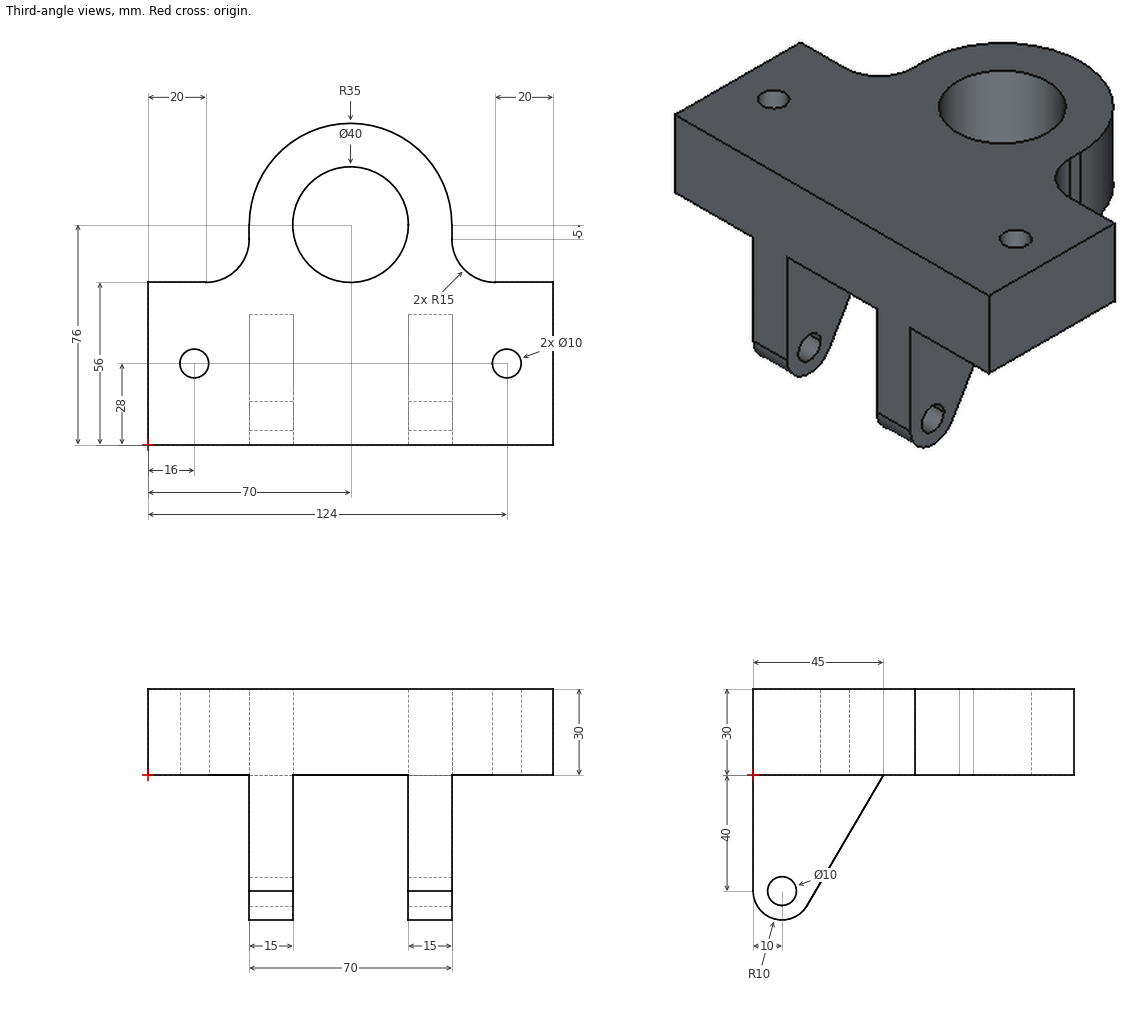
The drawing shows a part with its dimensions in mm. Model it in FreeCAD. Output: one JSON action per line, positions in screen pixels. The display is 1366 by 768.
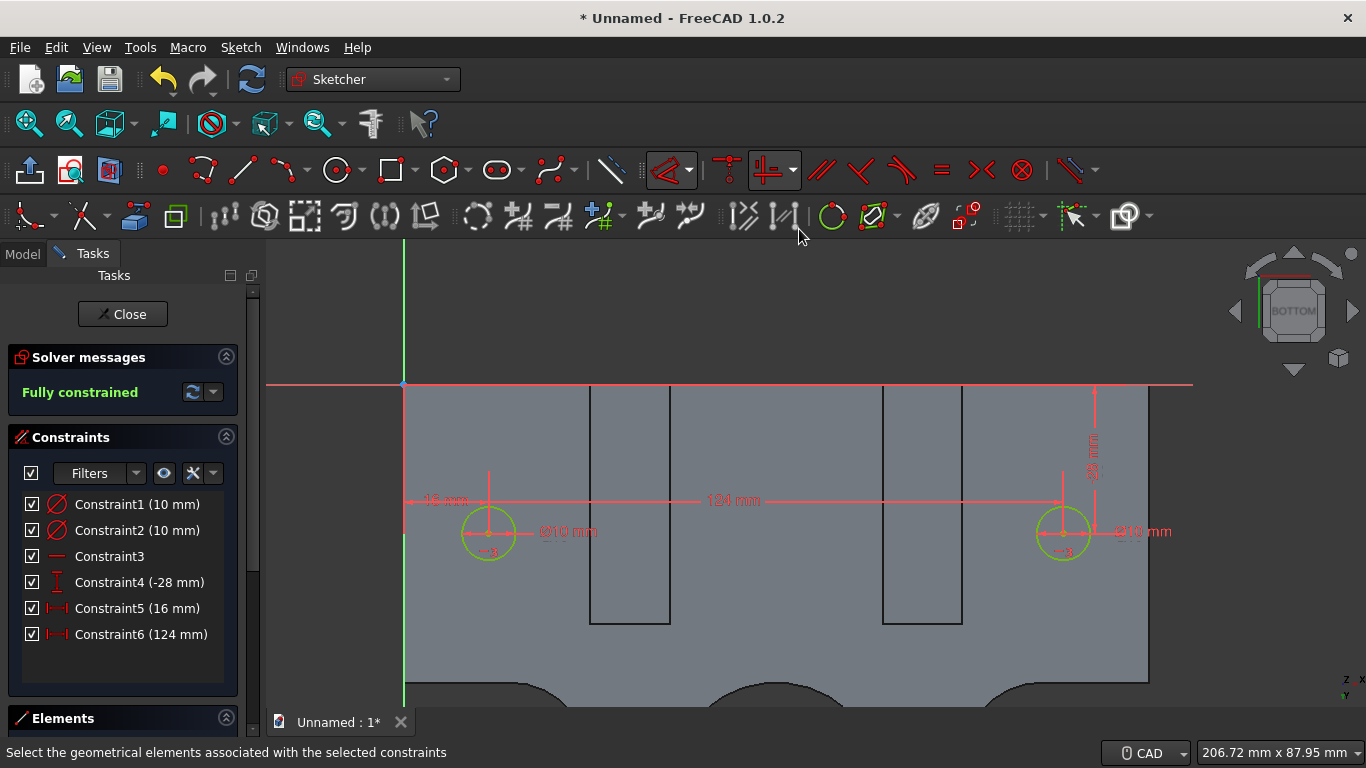
{"action": "left_click", "coordinate": [123, 314]}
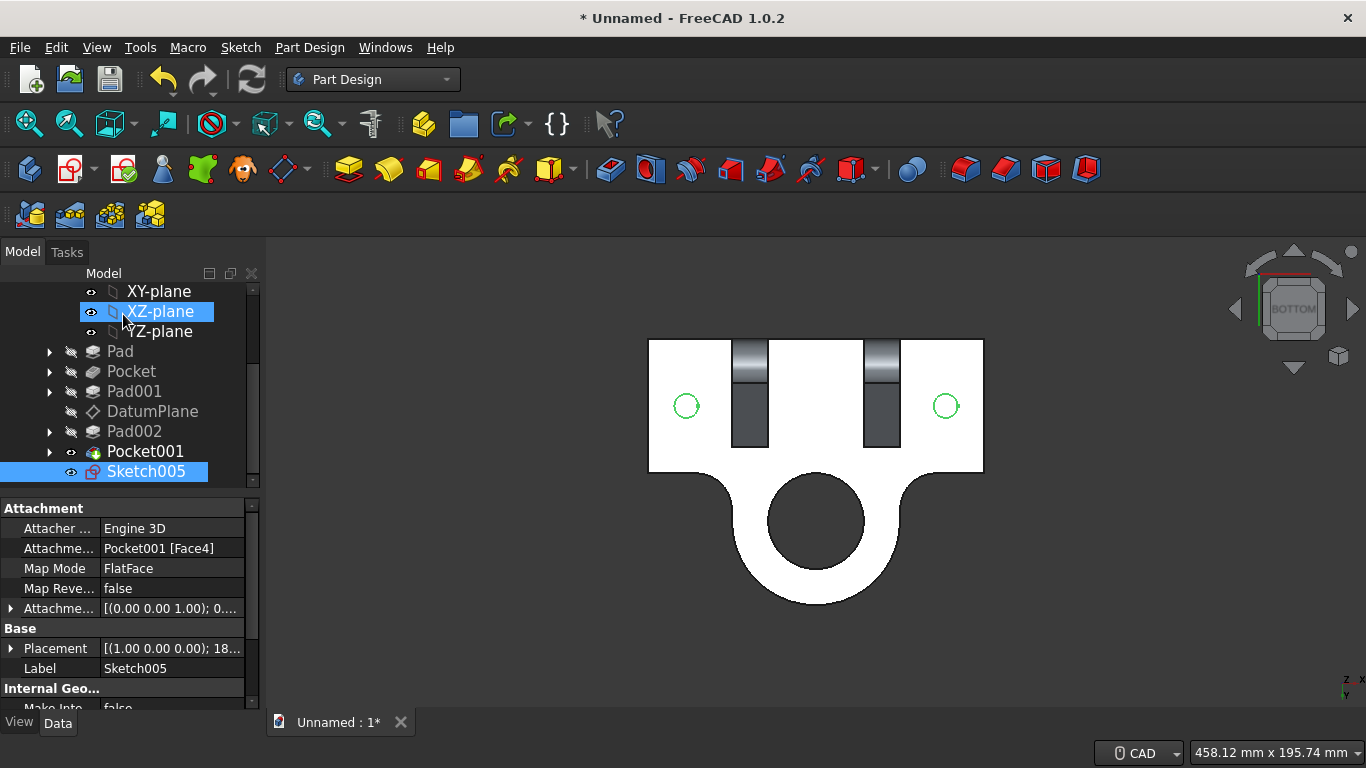
{"action": "left_click", "coordinate": [612, 170]}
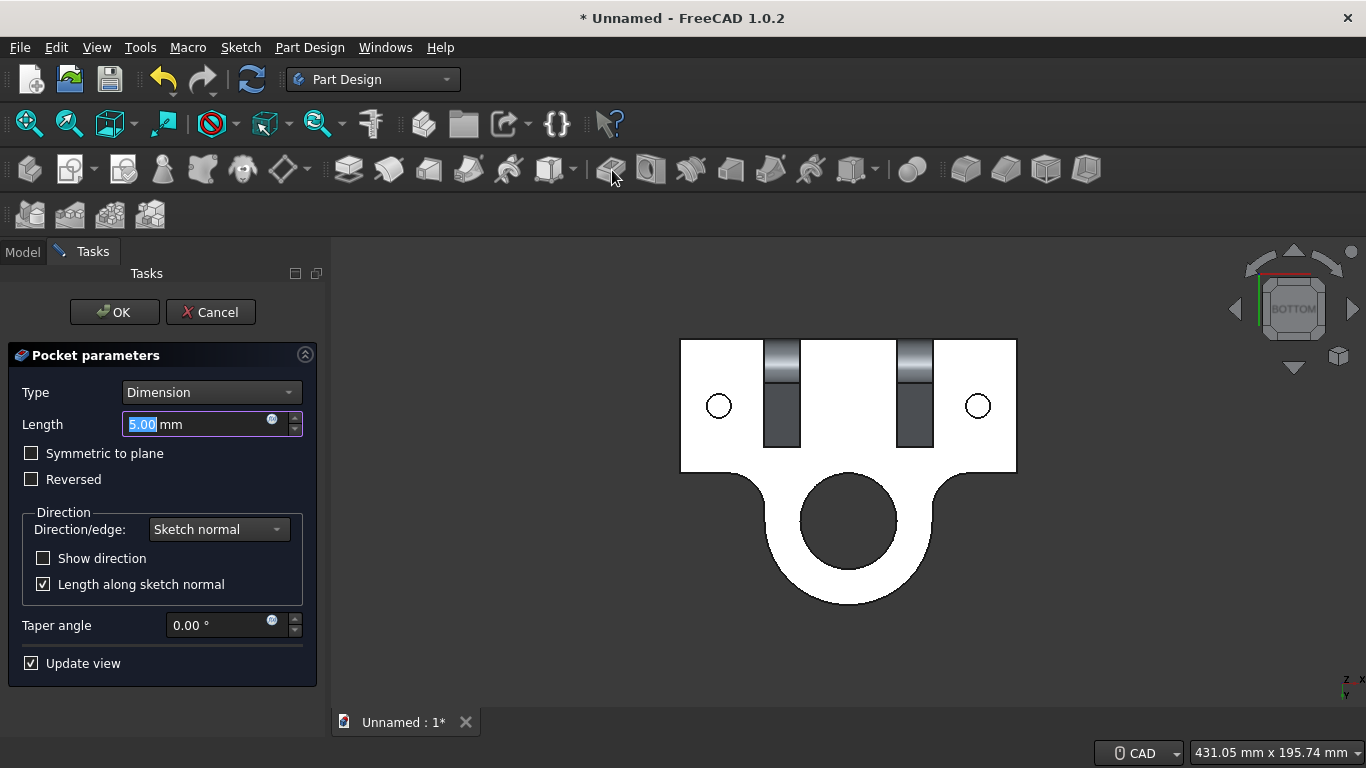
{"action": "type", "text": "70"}
{"action": "key", "text": "Tab"}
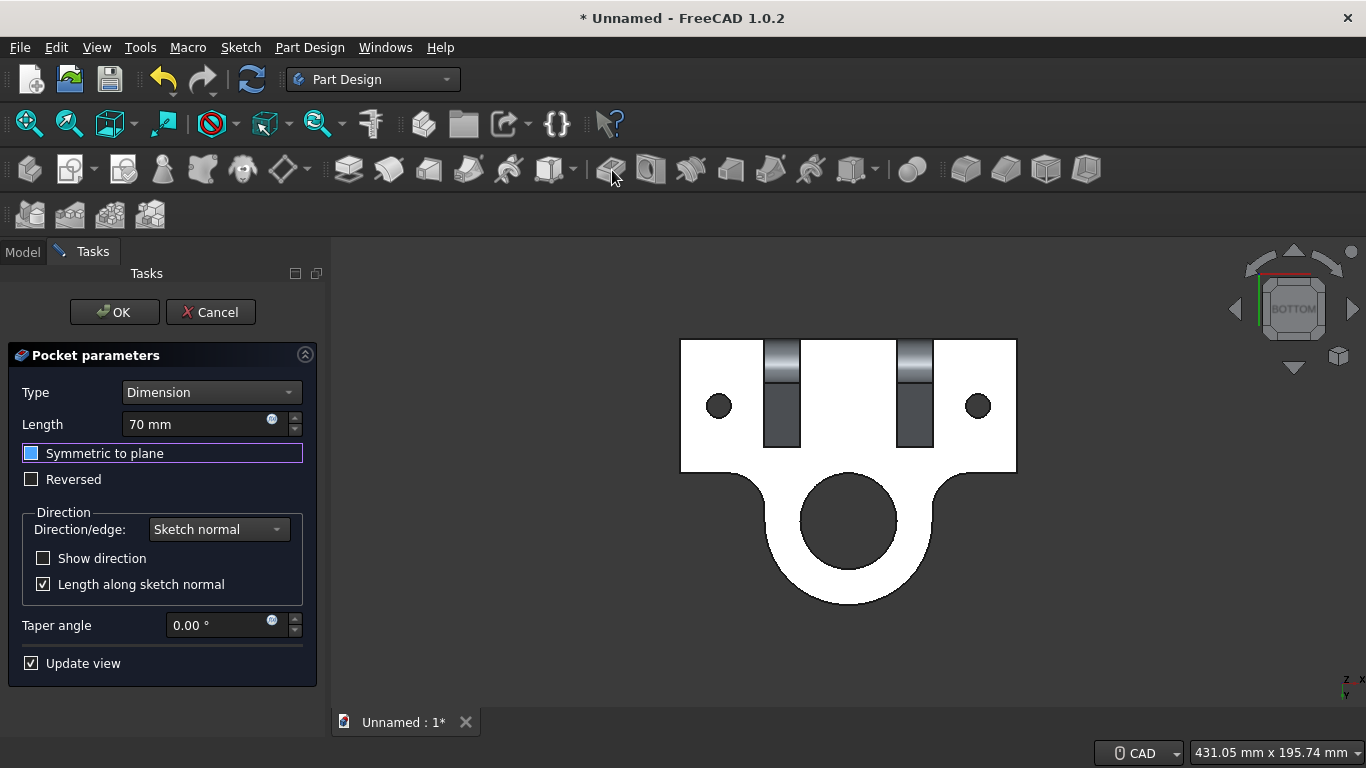
{"action": "left_click", "coordinate": [115, 312]}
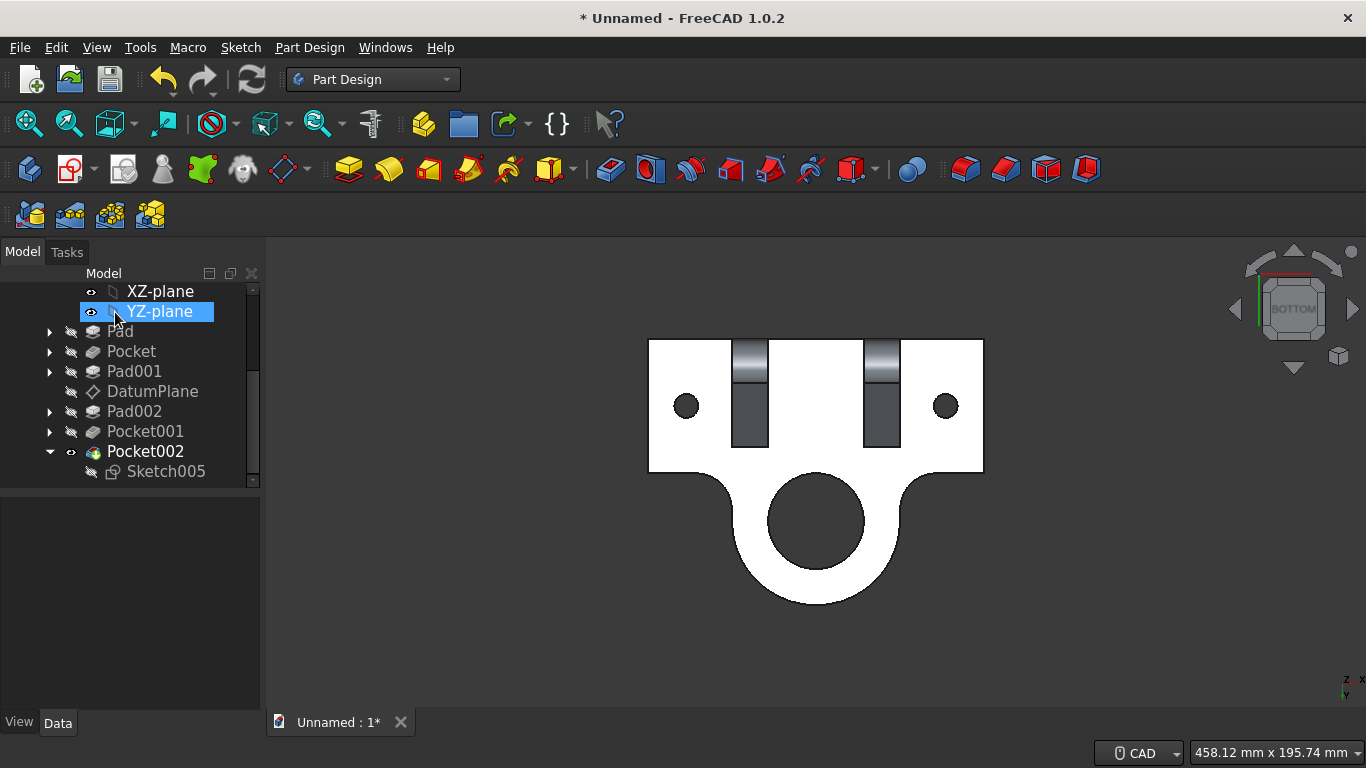
{"action": "key", "text": "0"}